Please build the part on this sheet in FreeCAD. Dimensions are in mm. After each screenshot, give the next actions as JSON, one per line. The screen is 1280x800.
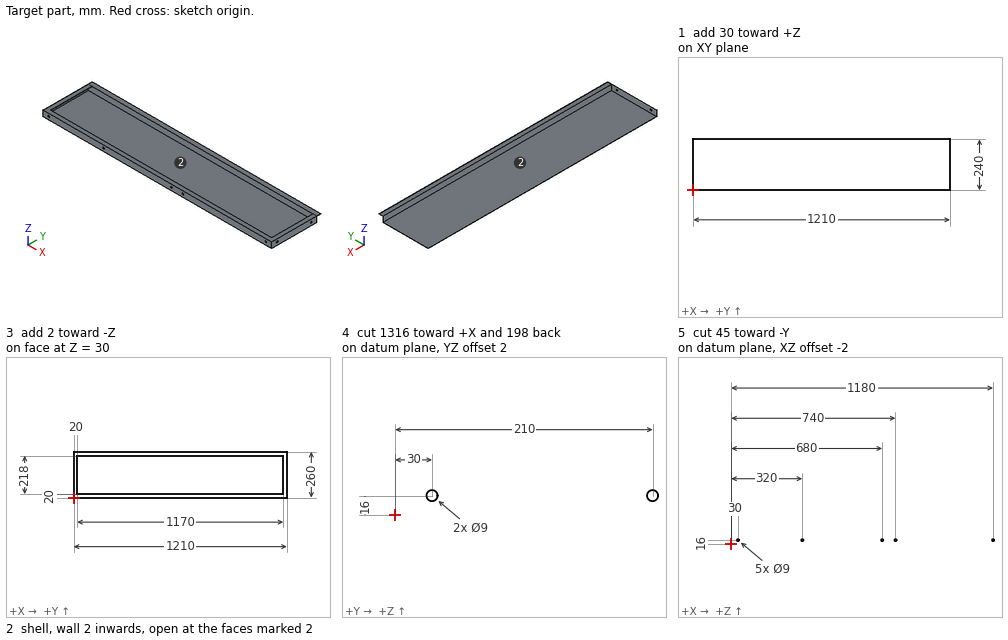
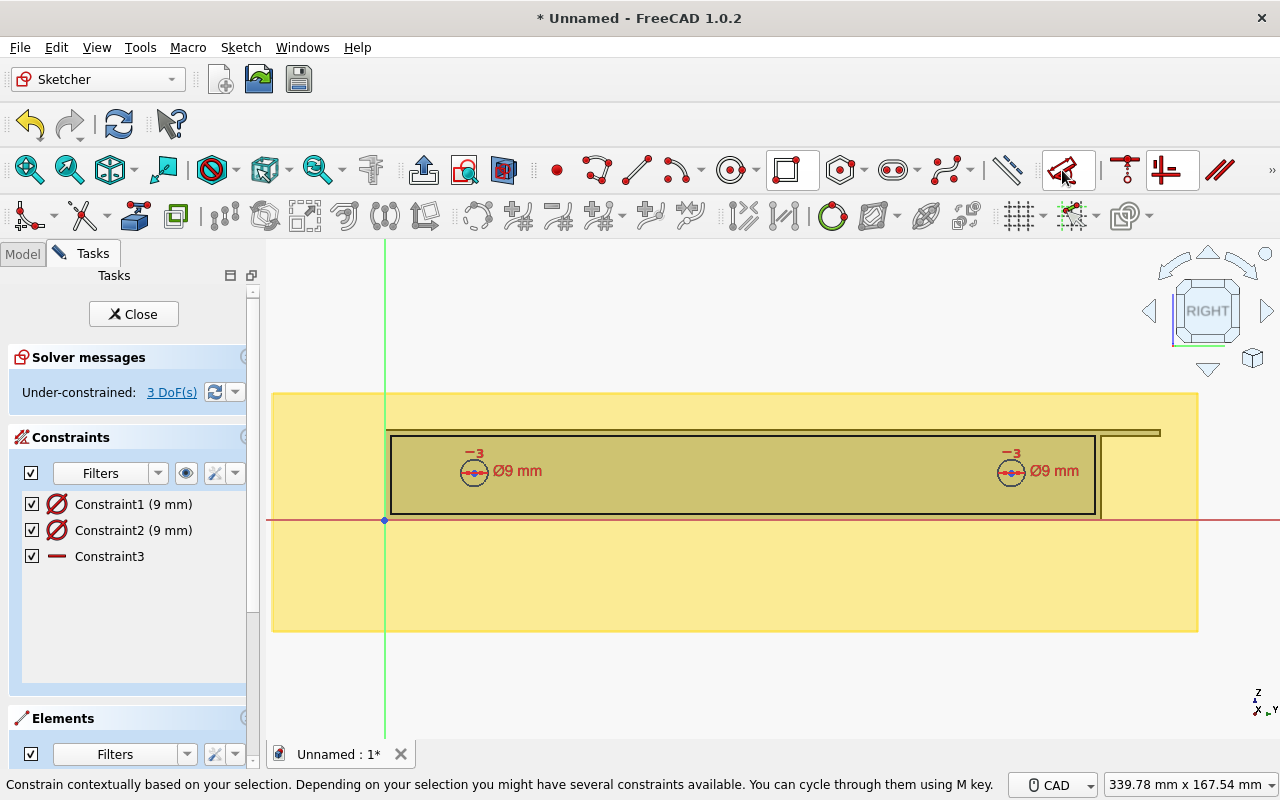
{"action": "left_click", "coordinate": [474, 473]}
{"action": "left_click", "coordinate": [429, 554]}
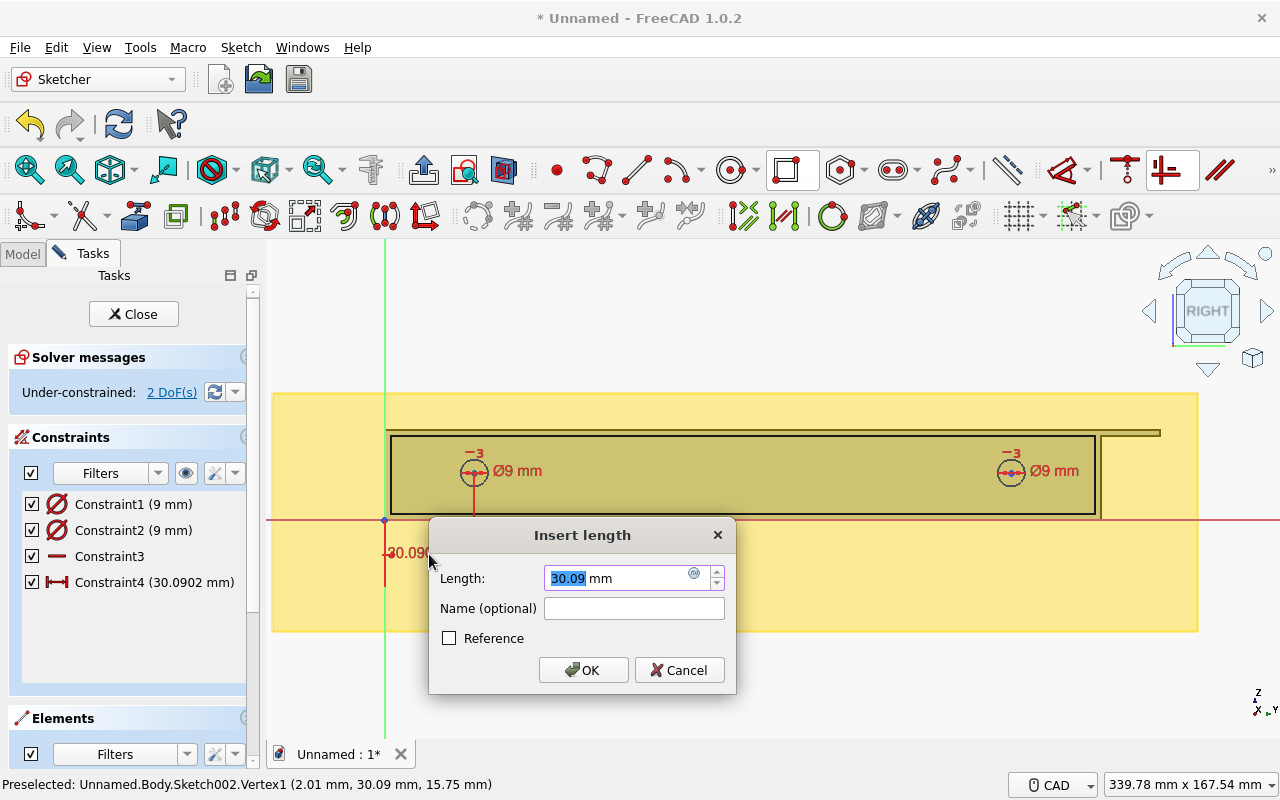
{"action": "type", "text": "30"}
{"action": "key", "text": "Return"}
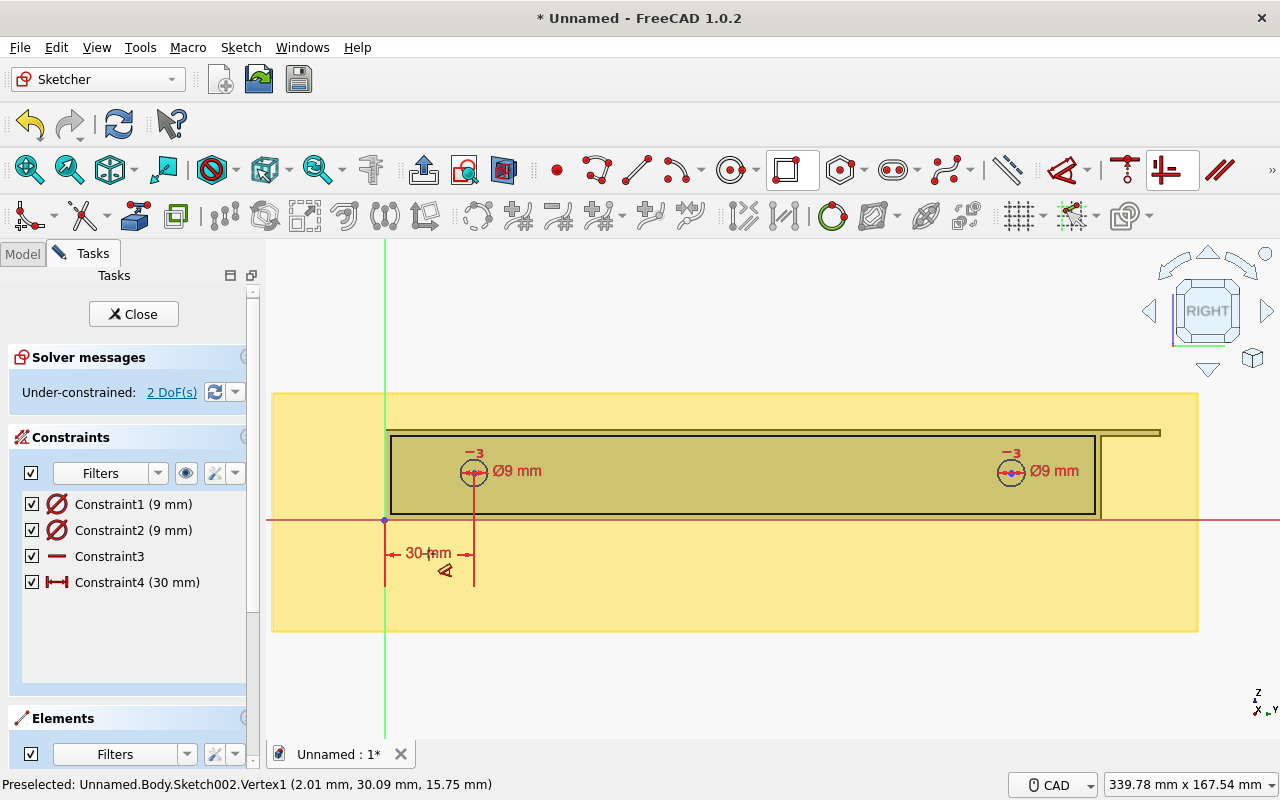
{"action": "left_click", "coordinate": [474, 473]}
{"action": "left_click", "coordinate": [351, 497]}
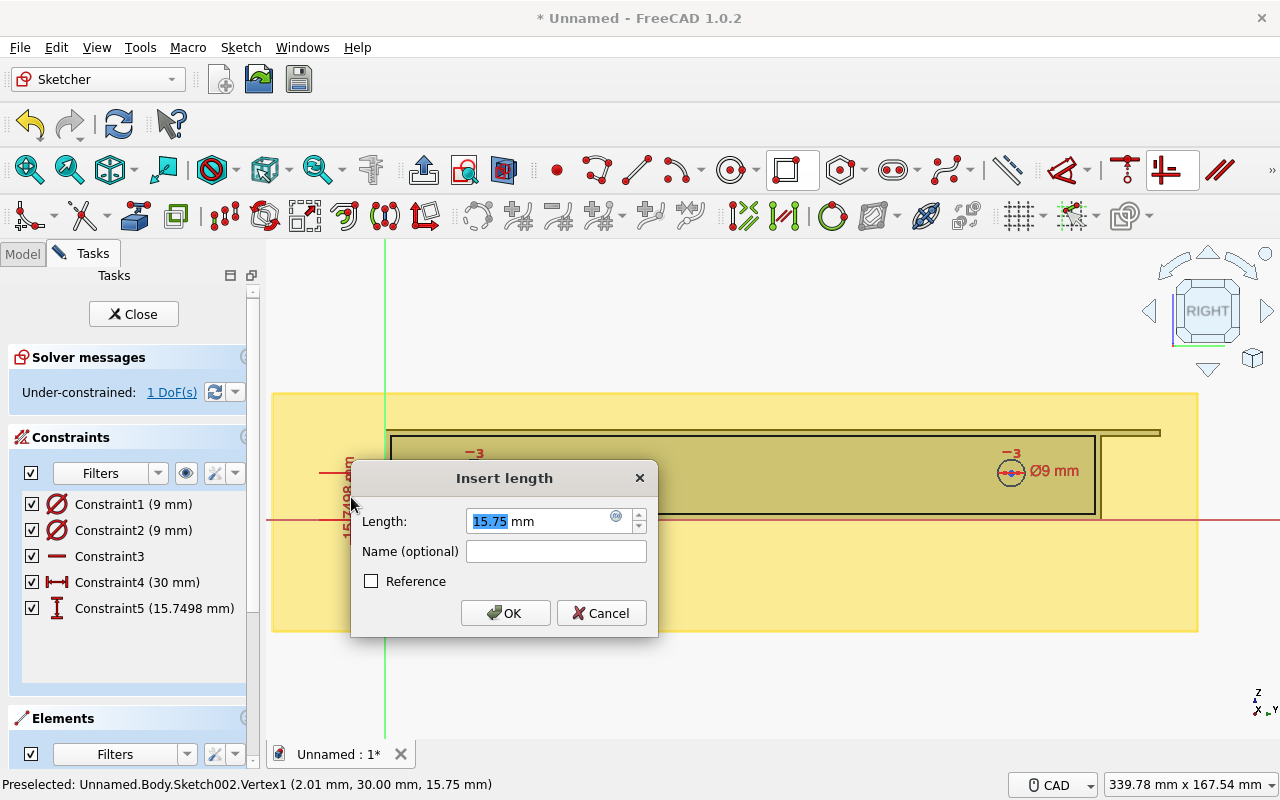
{"action": "type", "text": "16"}
{"action": "key", "text": "Return"}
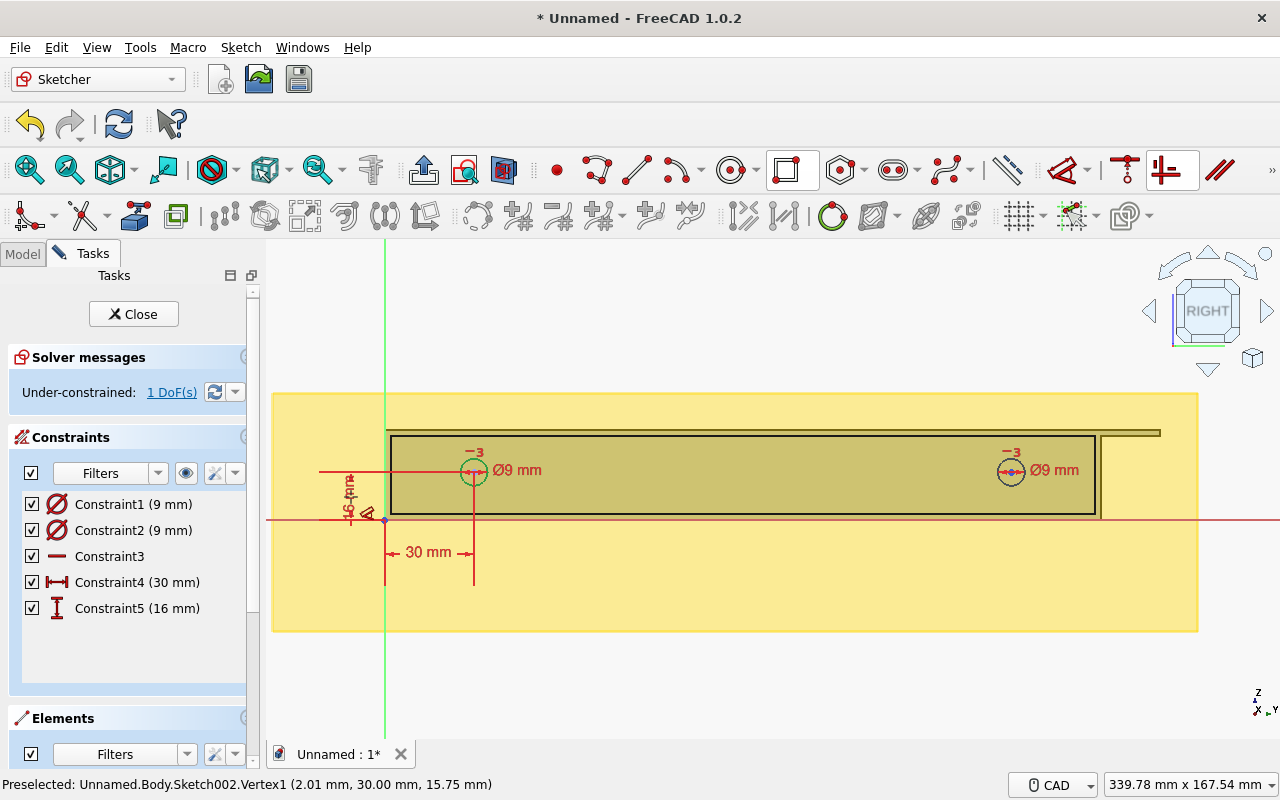
{"action": "left_click", "coordinate": [1011, 472]}
{"action": "left_click", "coordinate": [698, 554]}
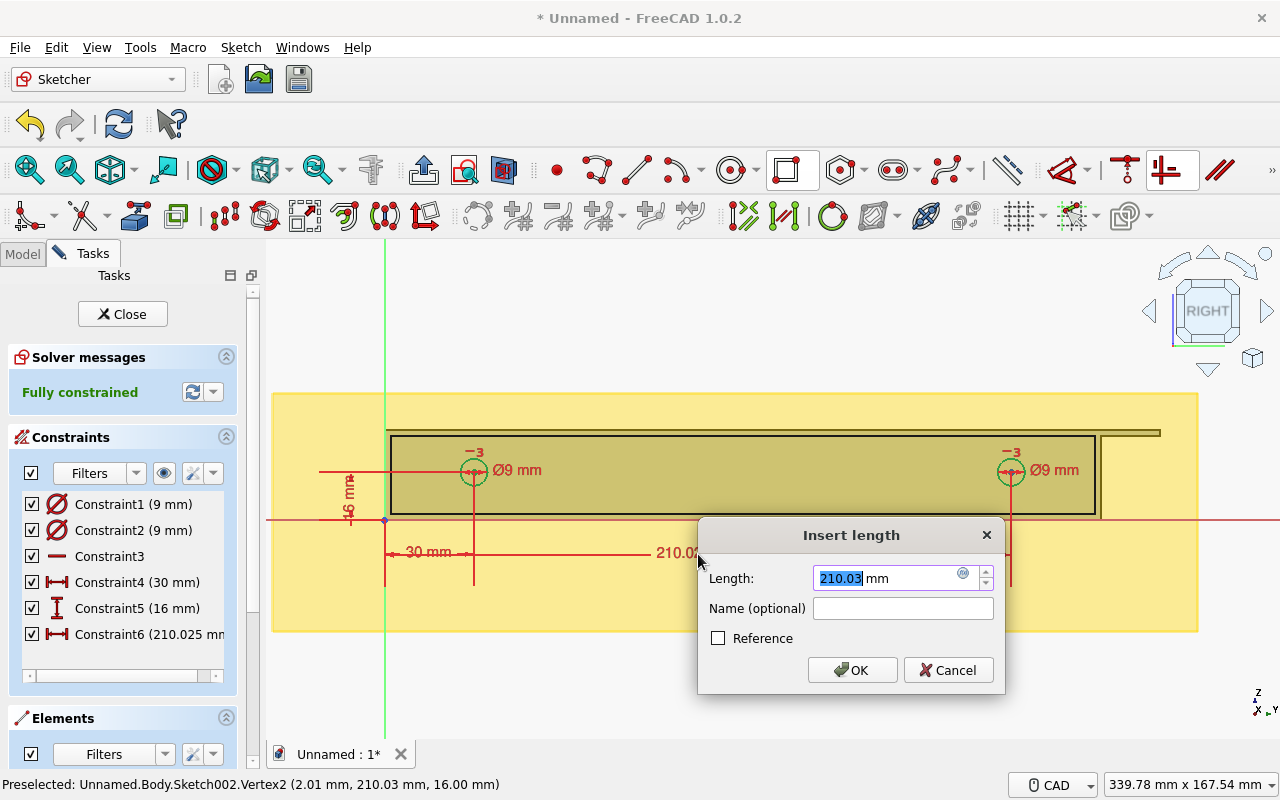
{"action": "type", "text": "210"}
{"action": "key", "text": "Return"}
{"action": "key", "text": "Escape"}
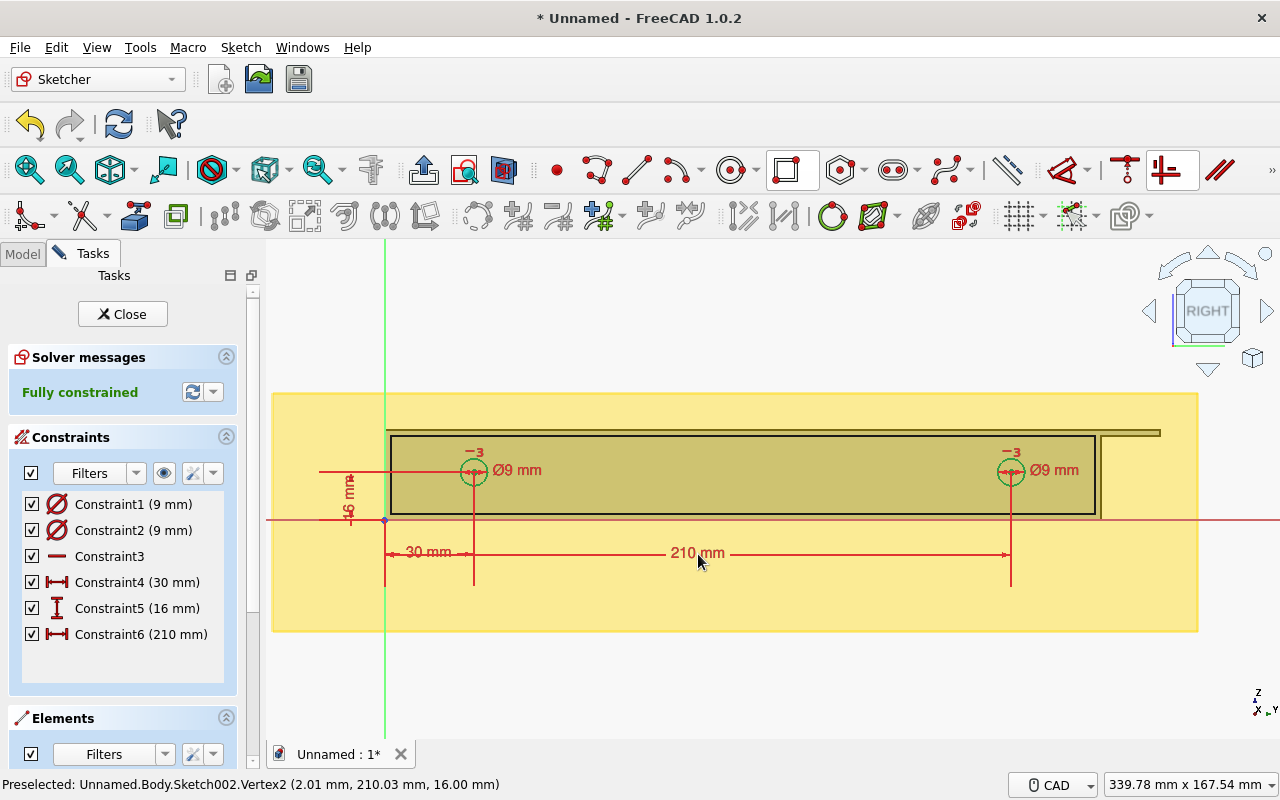
{"action": "left_click", "coordinate": [123, 314]}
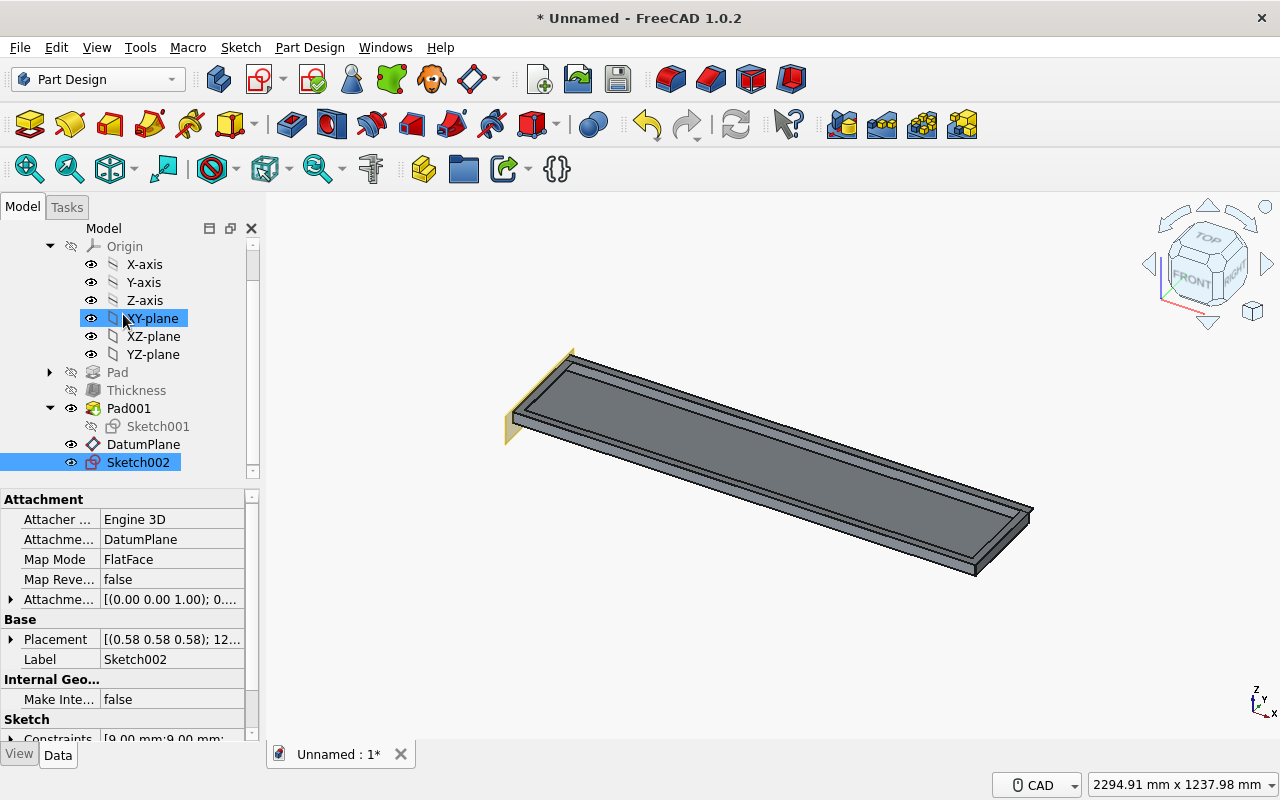
{"action": "left_click", "coordinate": [292, 124]}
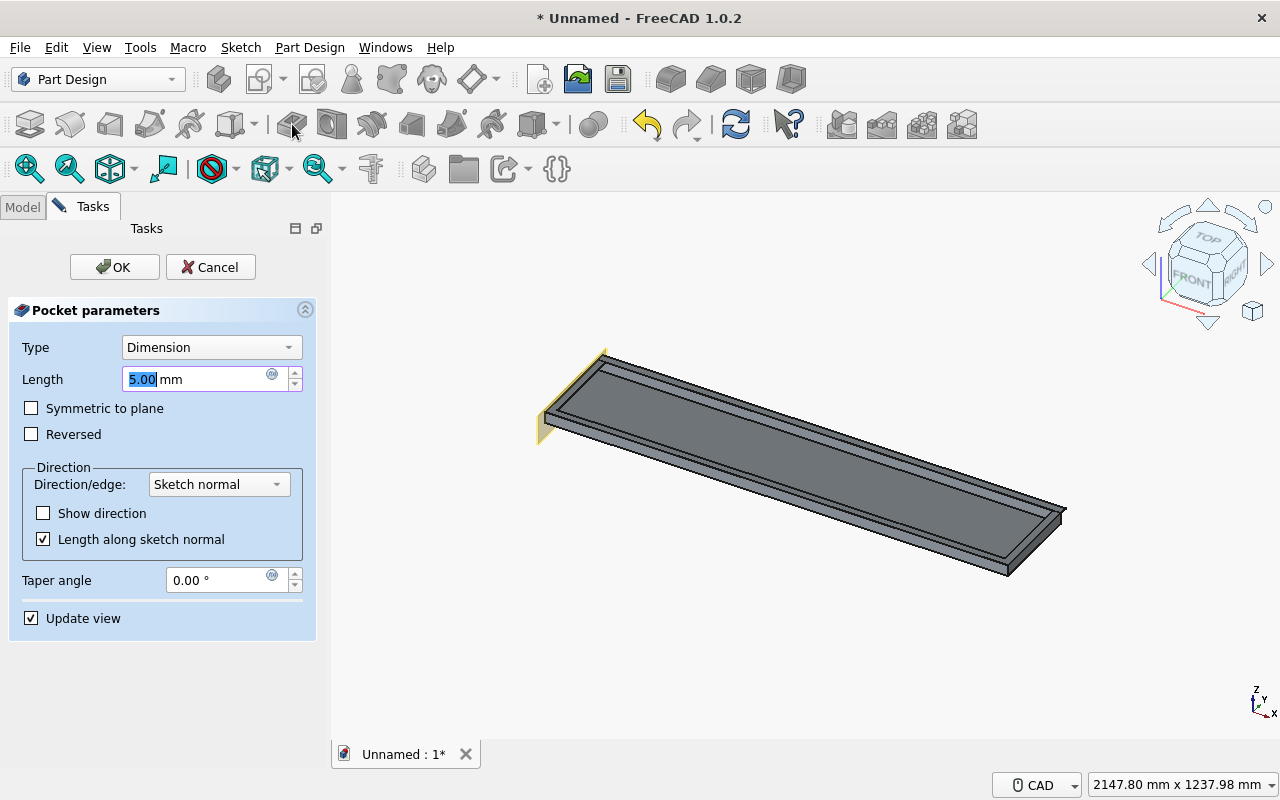
{"action": "left_click", "coordinate": [212, 348]}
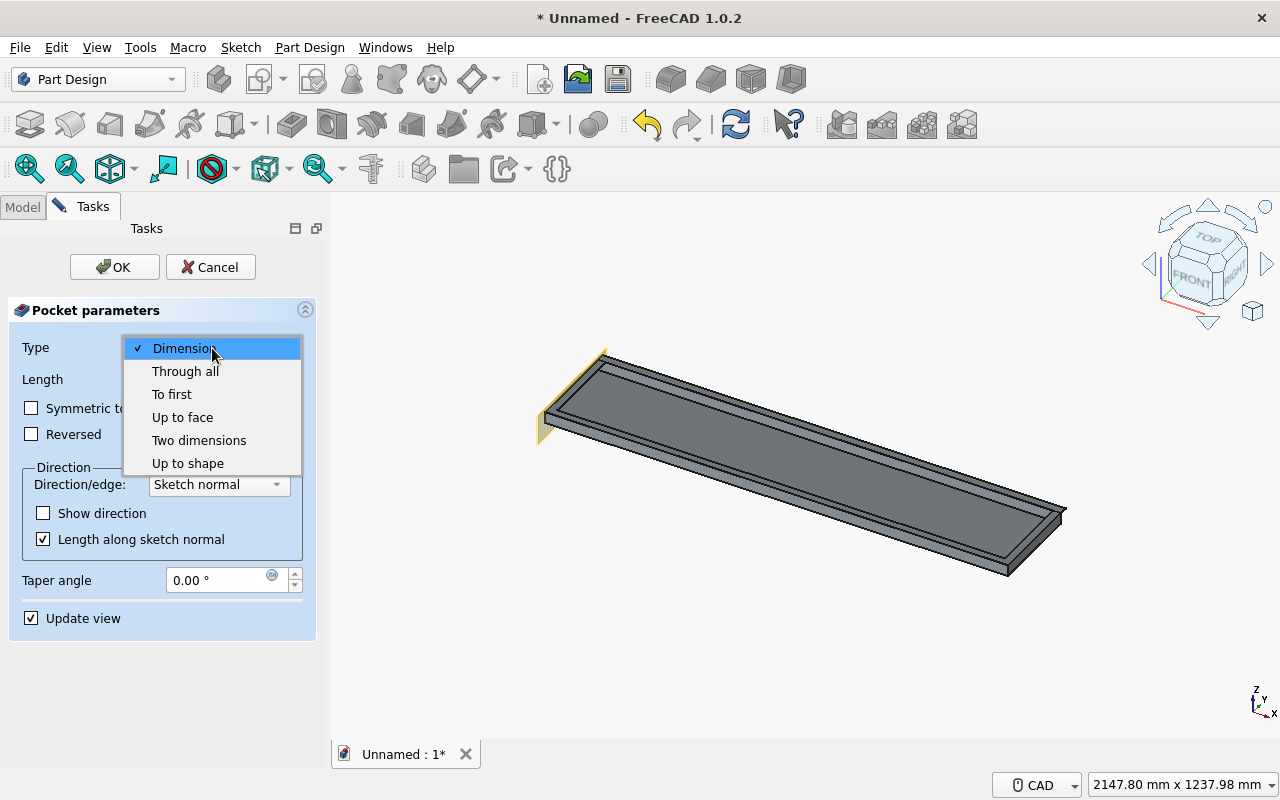
{"action": "left_click", "coordinate": [212, 440]}